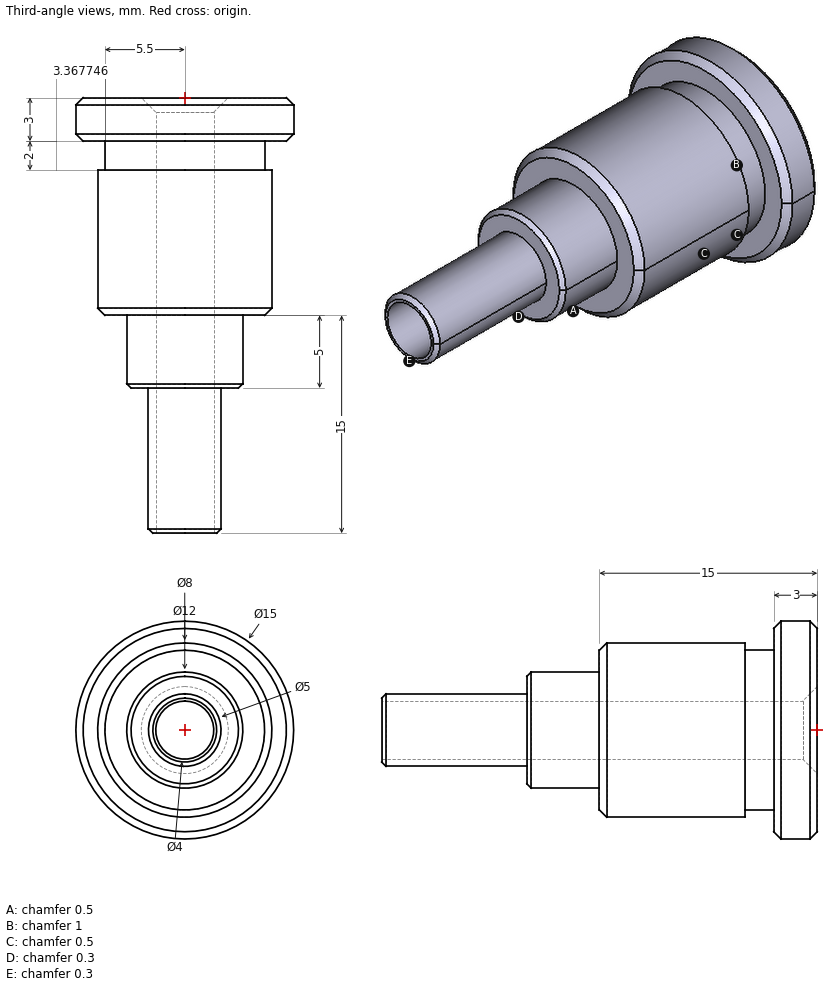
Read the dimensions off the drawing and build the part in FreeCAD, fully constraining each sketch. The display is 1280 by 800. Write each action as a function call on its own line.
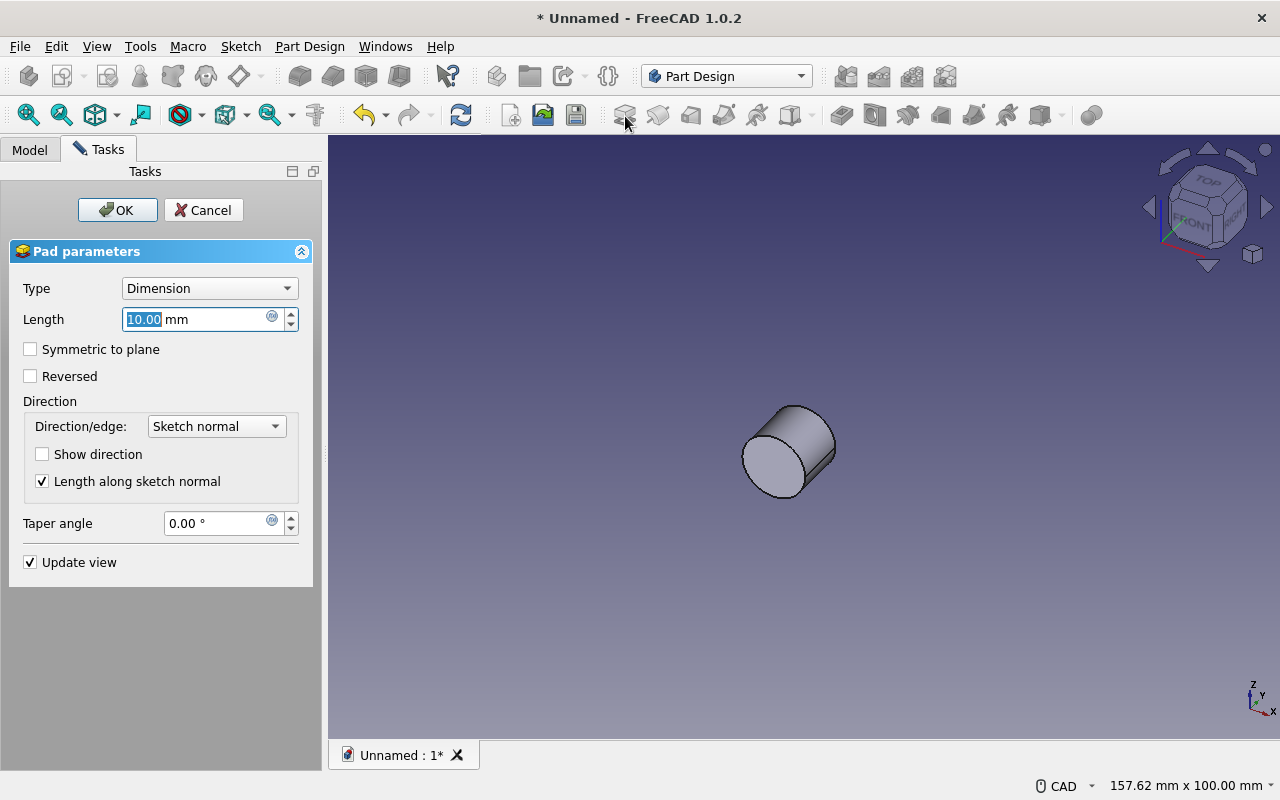
text(15)
key(Tab)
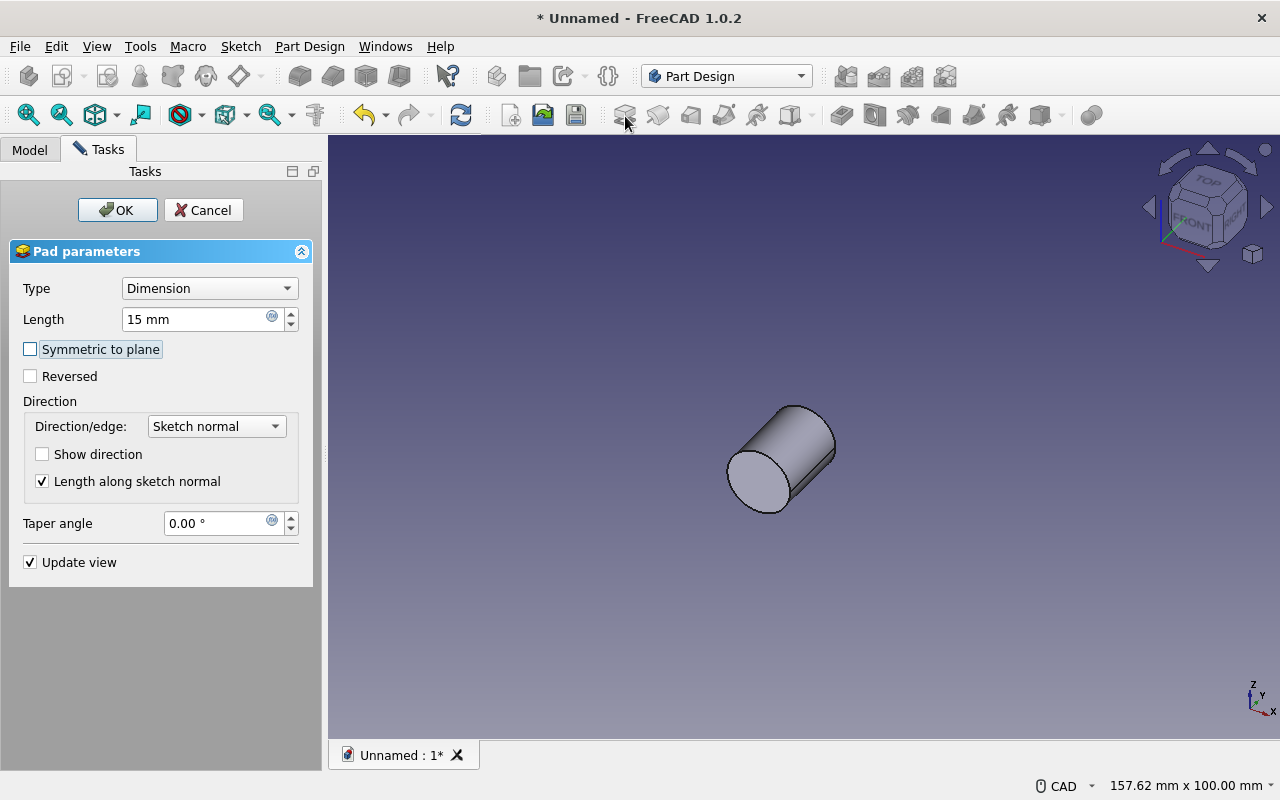
click(118, 210)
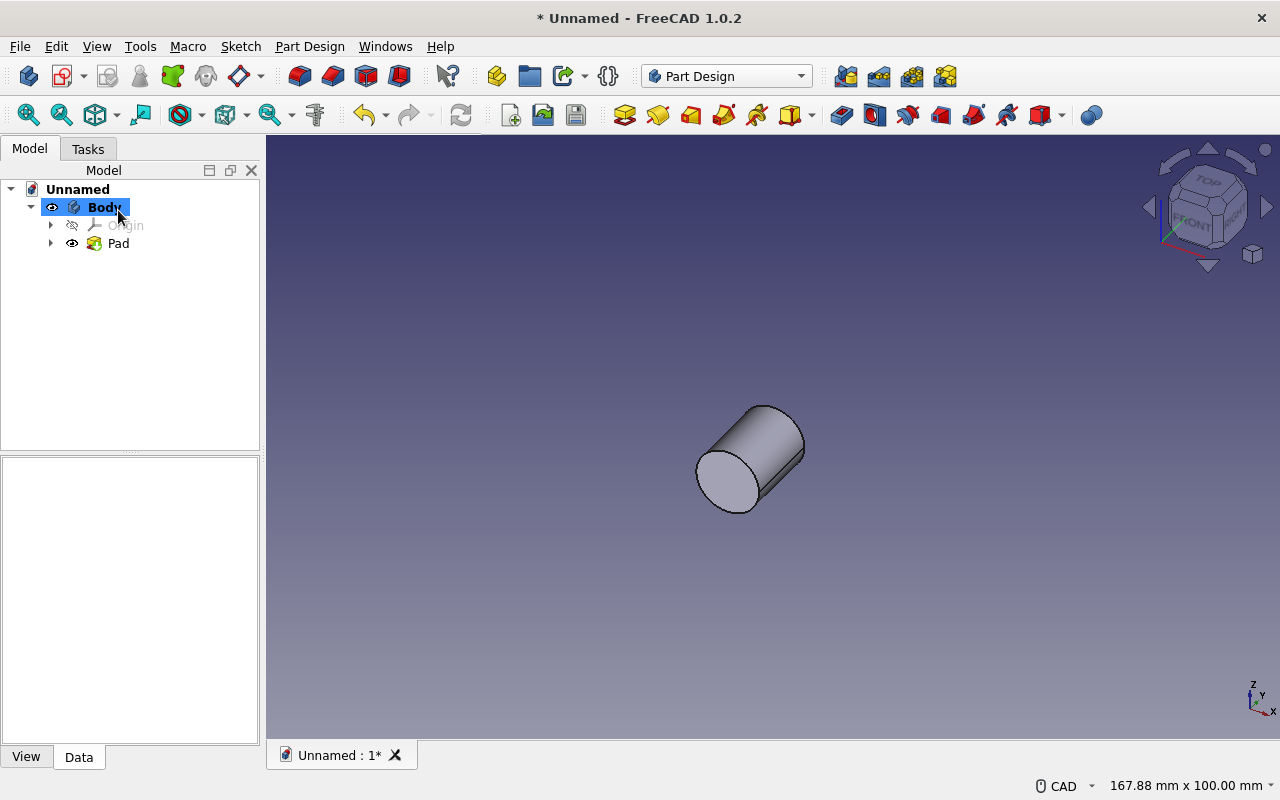
click(29, 116)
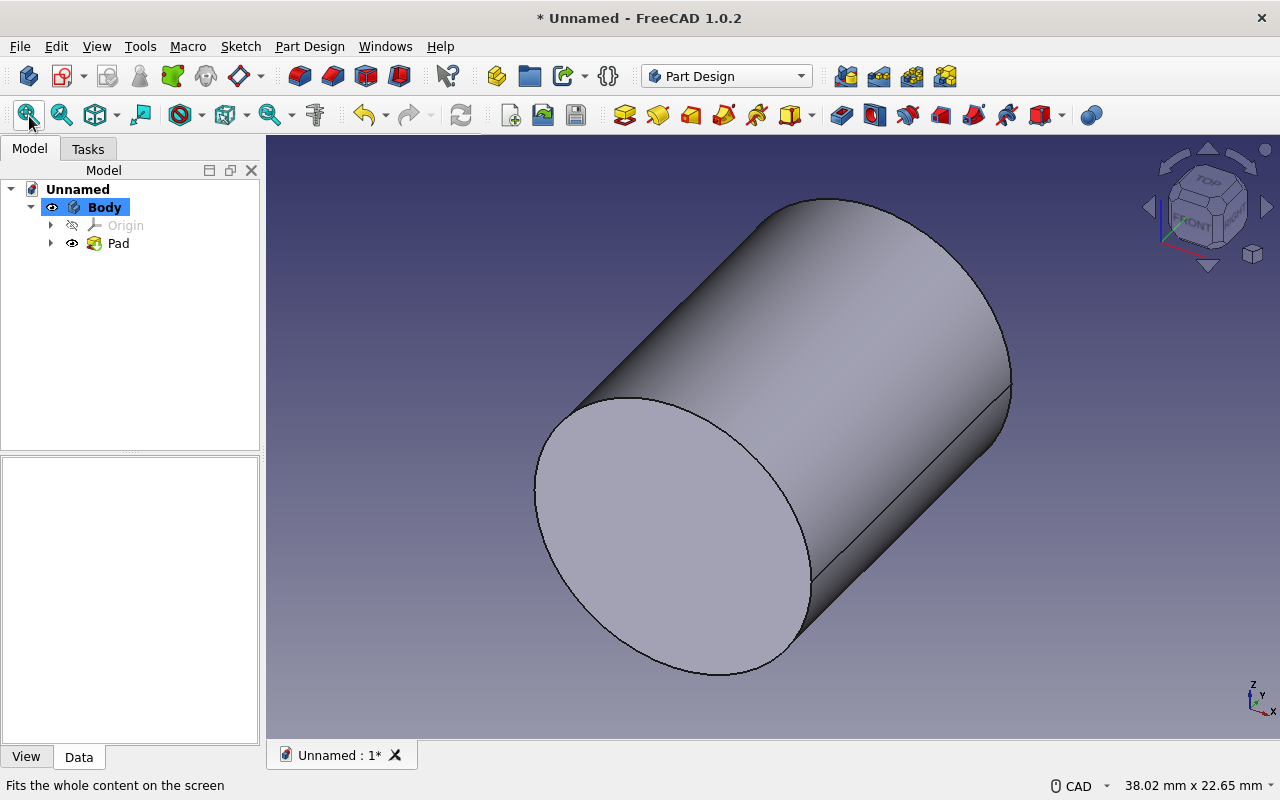
click(673, 535)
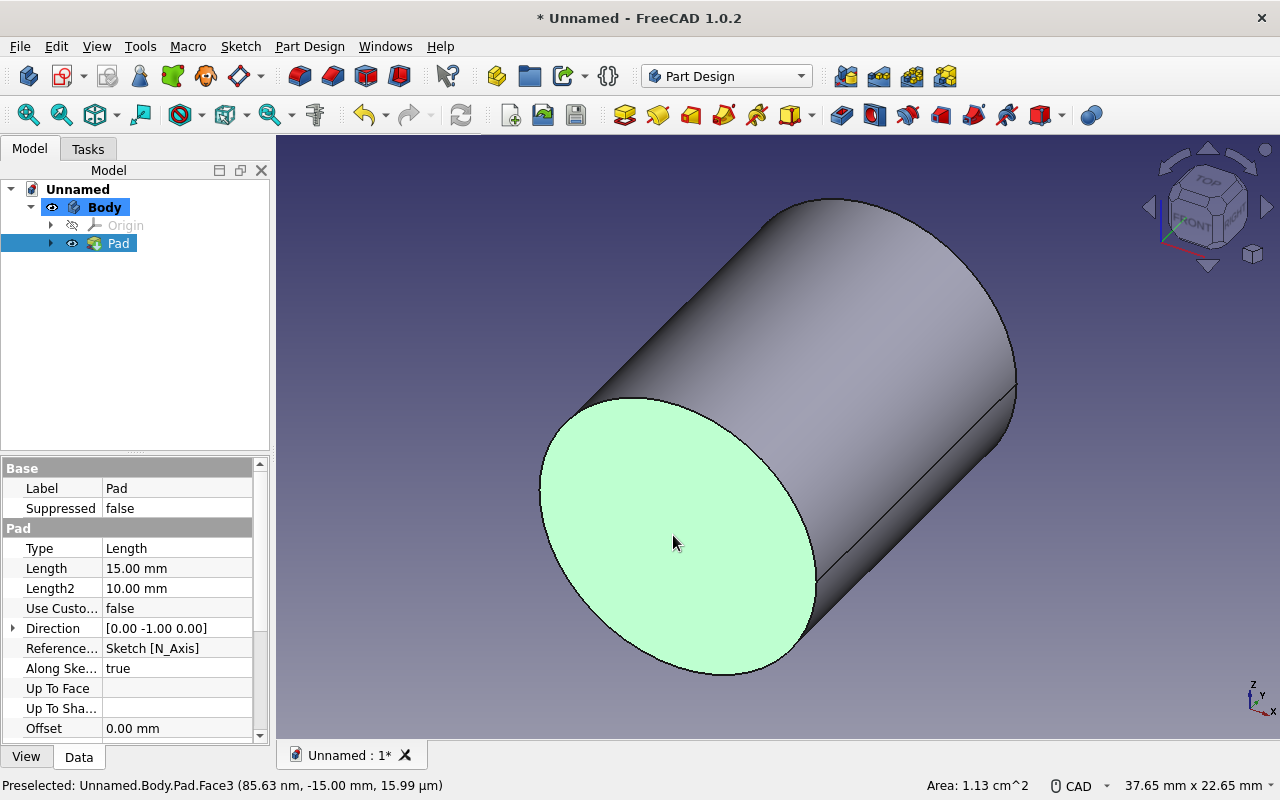
click(62, 76)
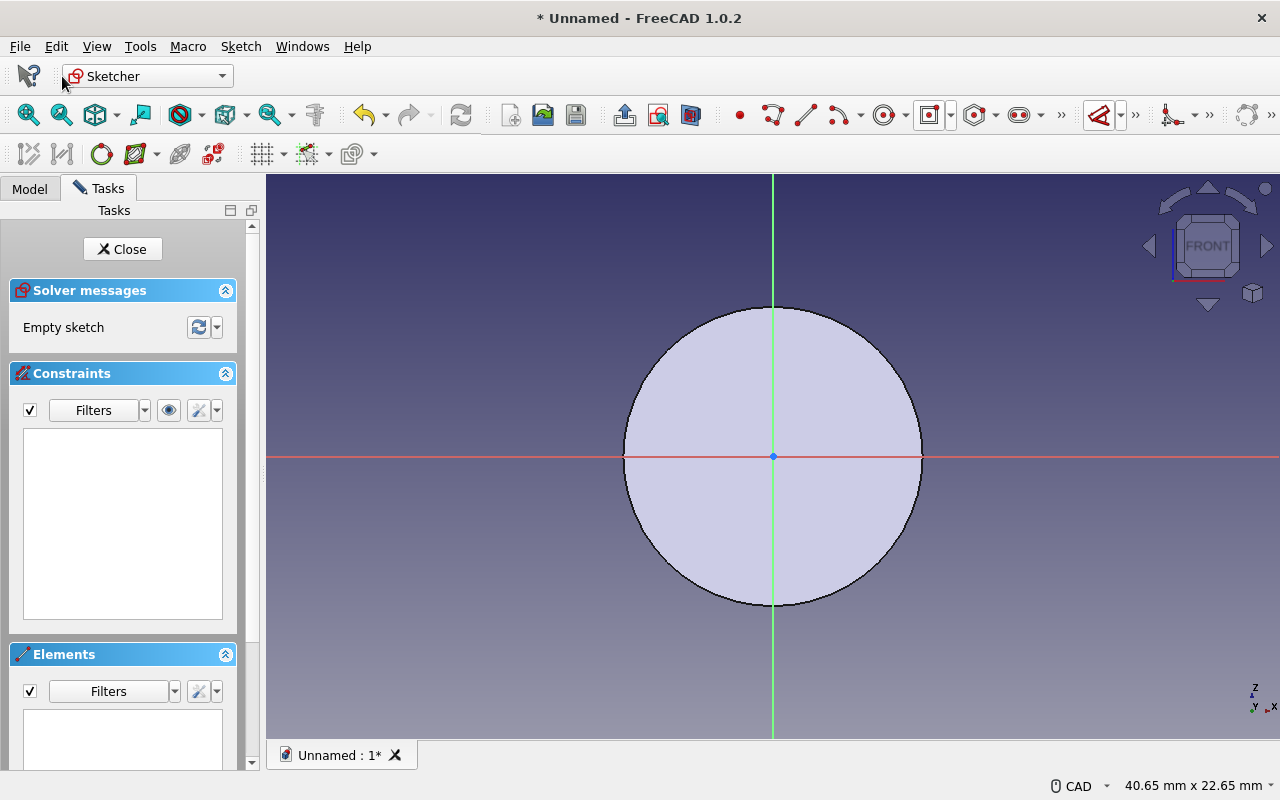
scroll(813, 456, up, 5)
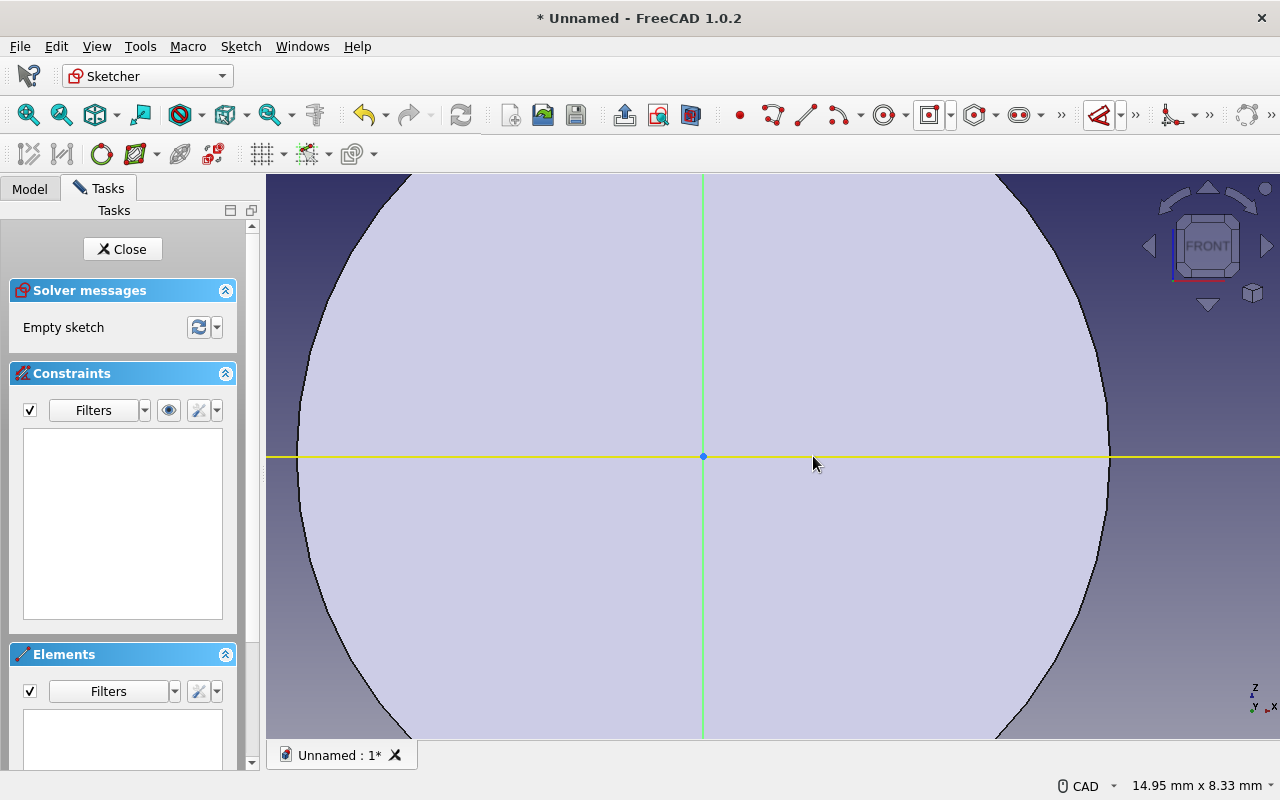
click(884, 116)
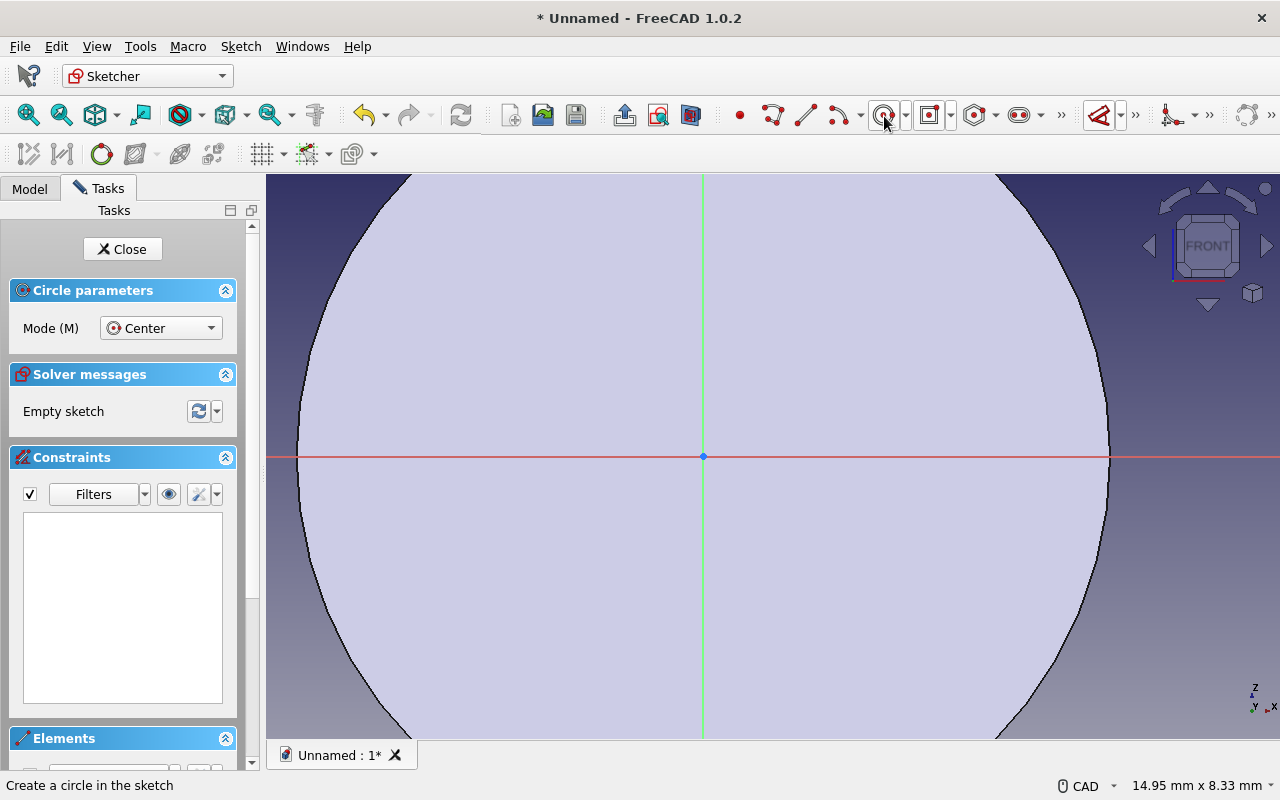
click(703, 456)
move(823, 337)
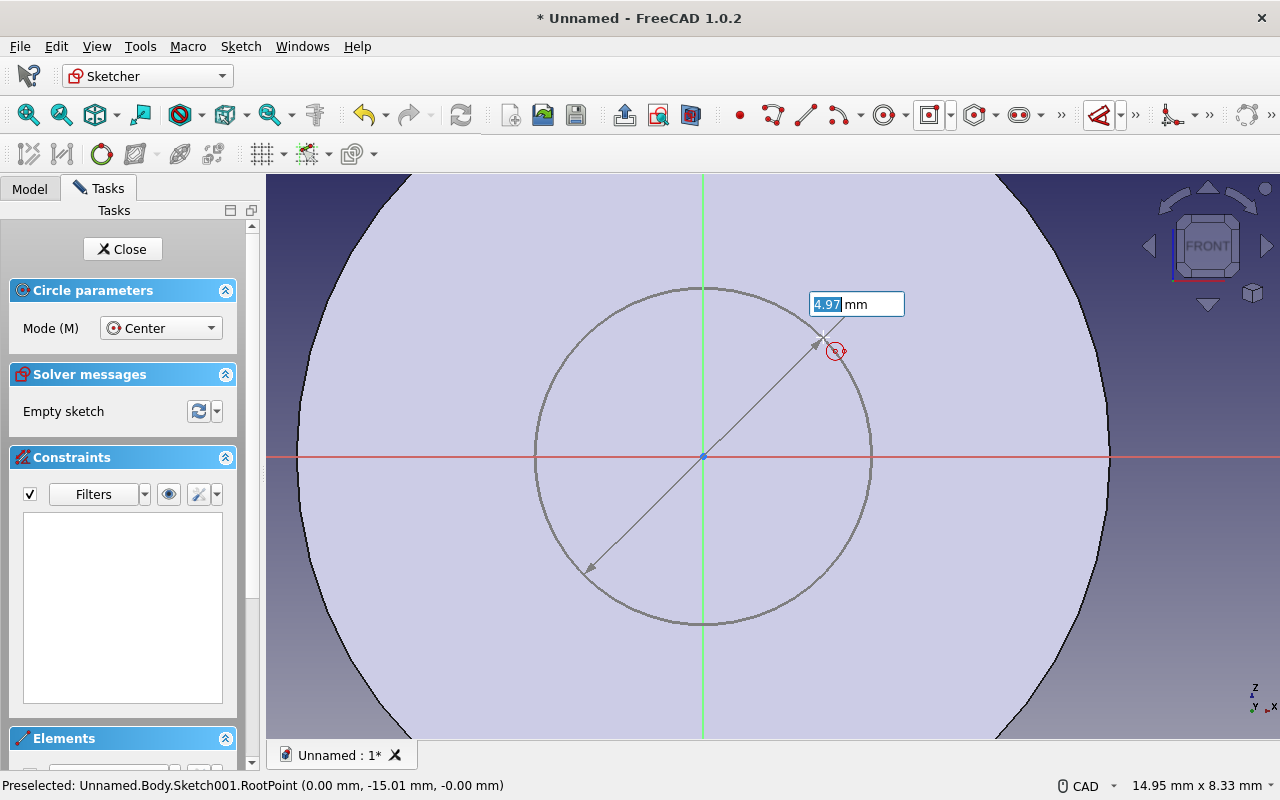
text(5)
key(Return)
key(Escape)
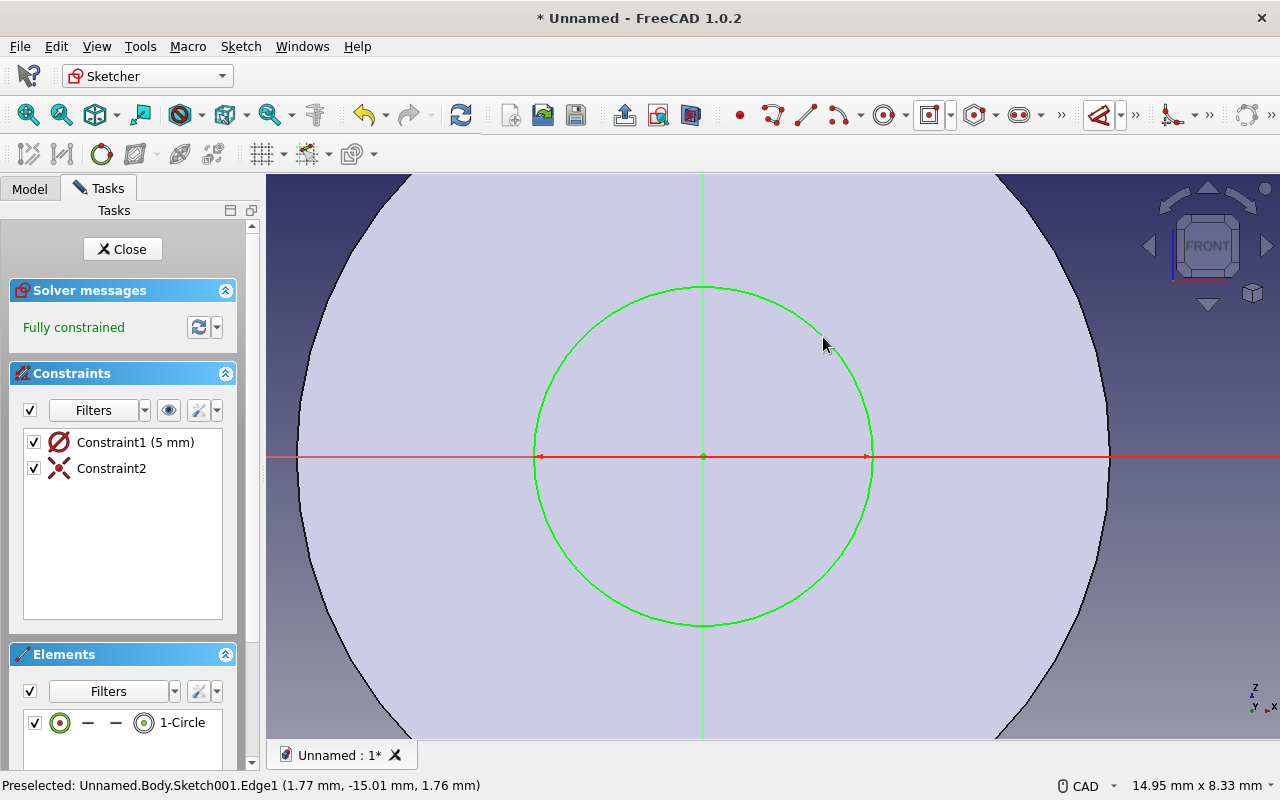
click(123, 249)